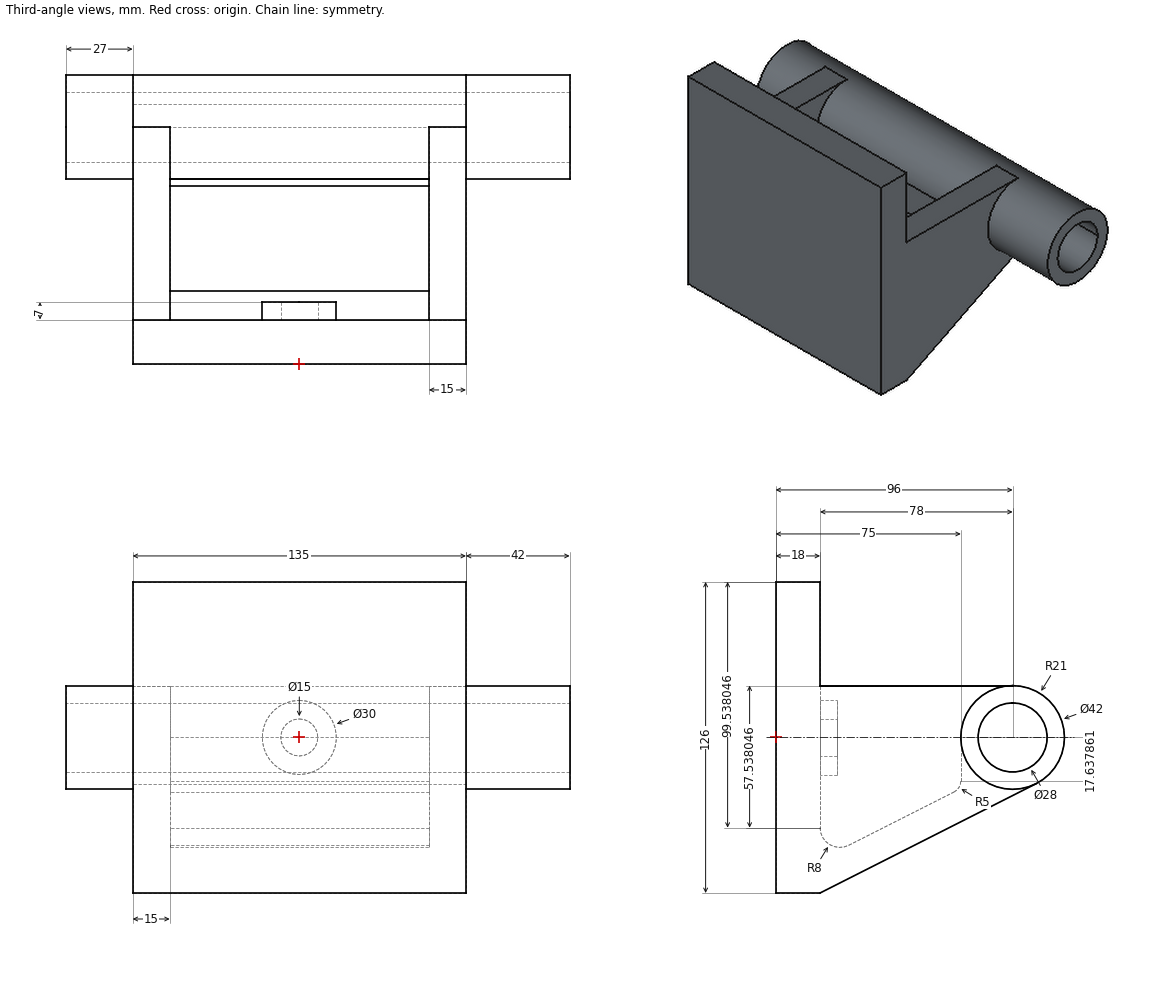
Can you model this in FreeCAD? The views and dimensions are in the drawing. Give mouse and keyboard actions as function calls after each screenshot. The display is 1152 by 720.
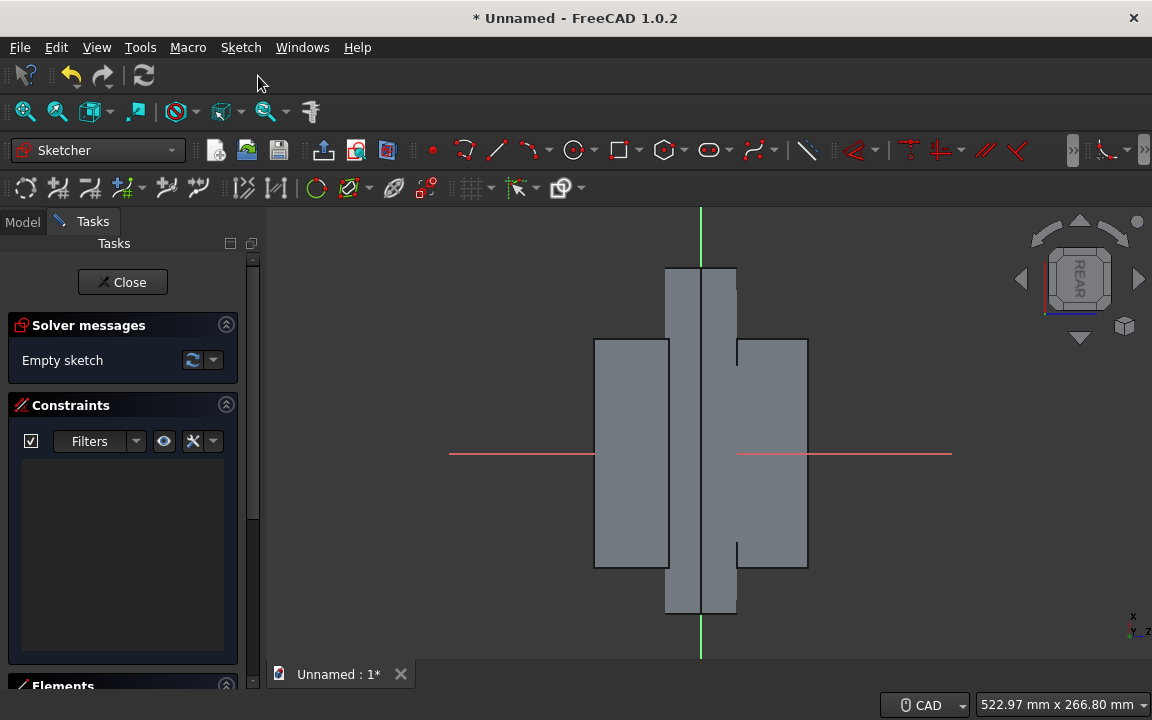
scroll(713, 458, up, 9)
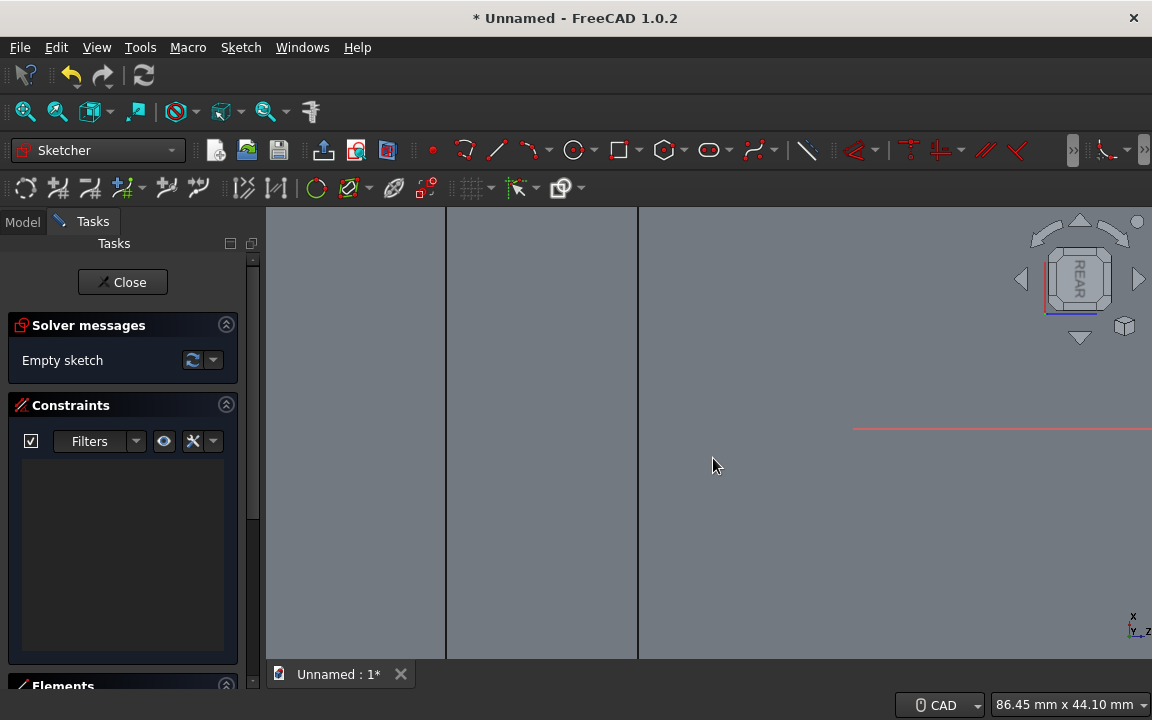
click(574, 150)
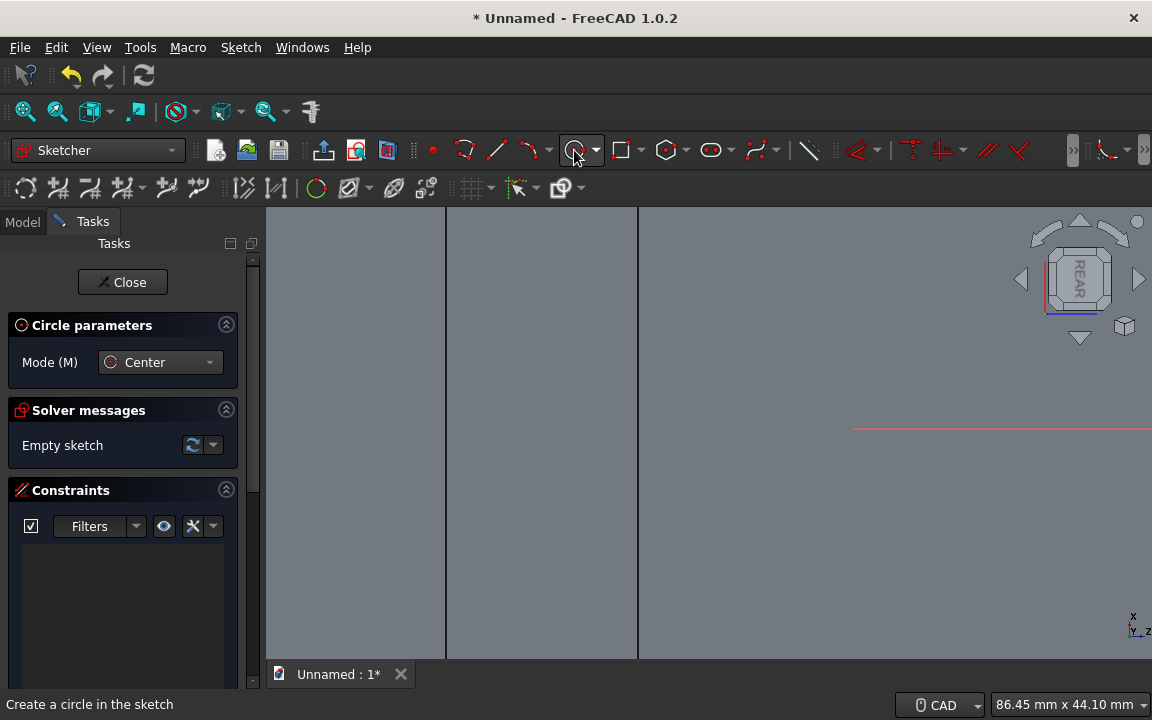
click(638, 429)
click(746, 321)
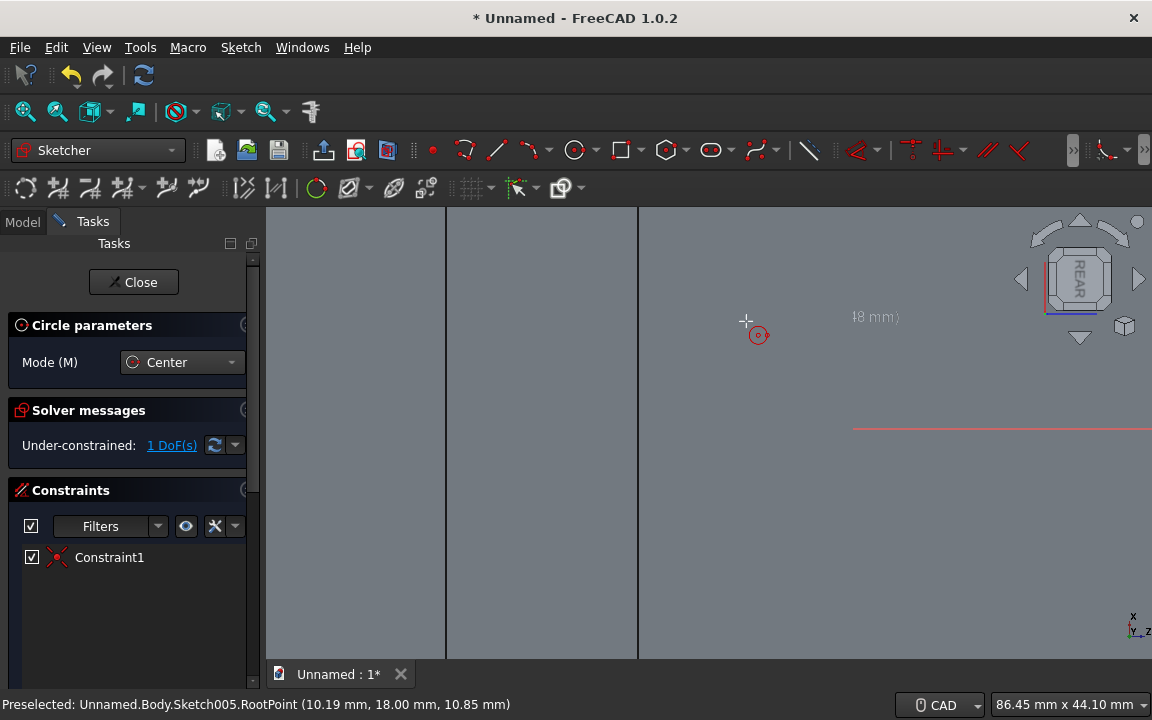
click(638, 429)
click(692, 375)
key(Escape)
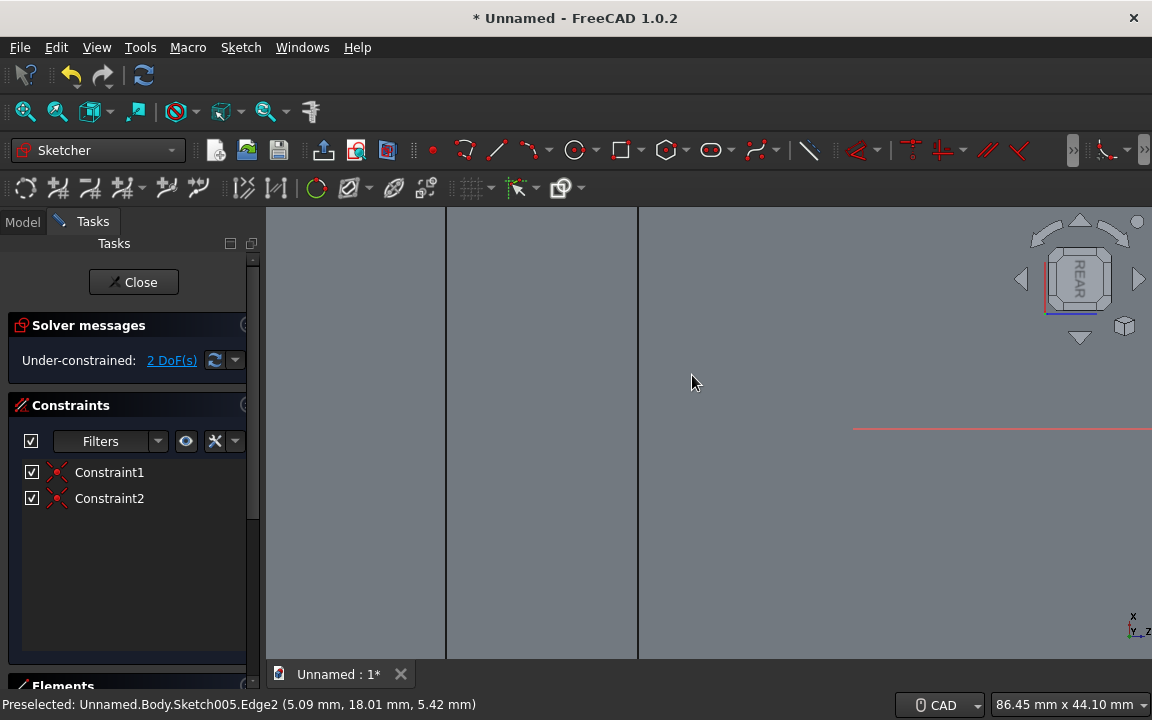
click(856, 150)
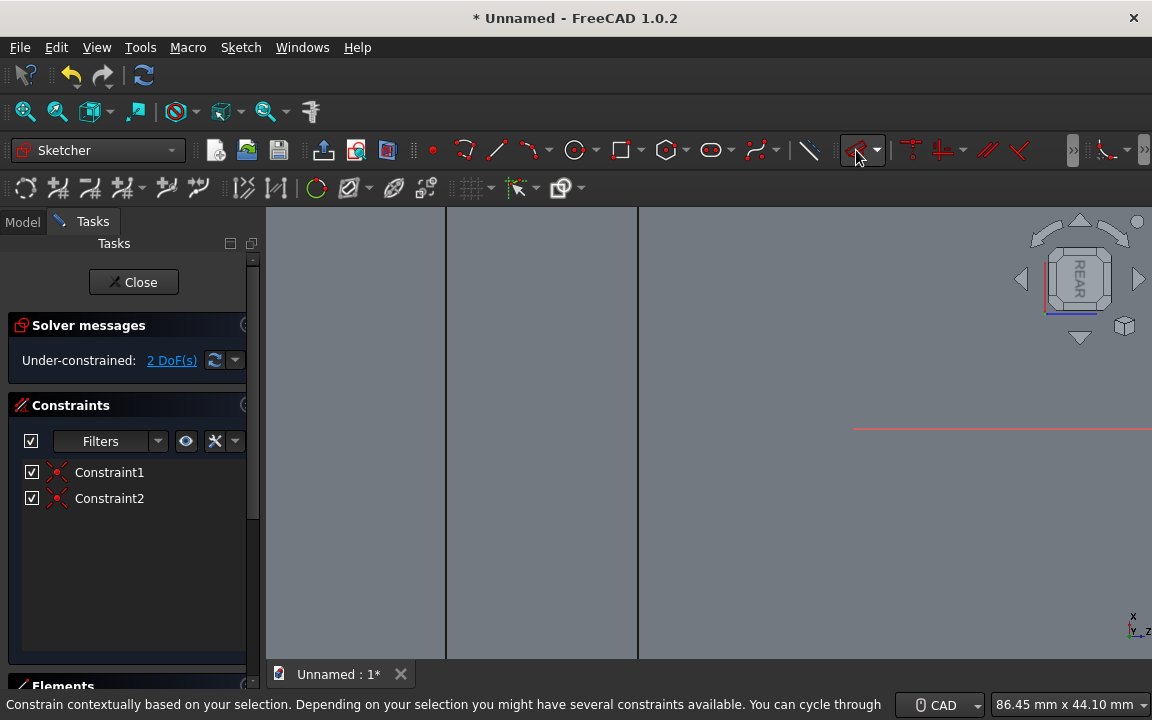
click(745, 321)
click(768, 298)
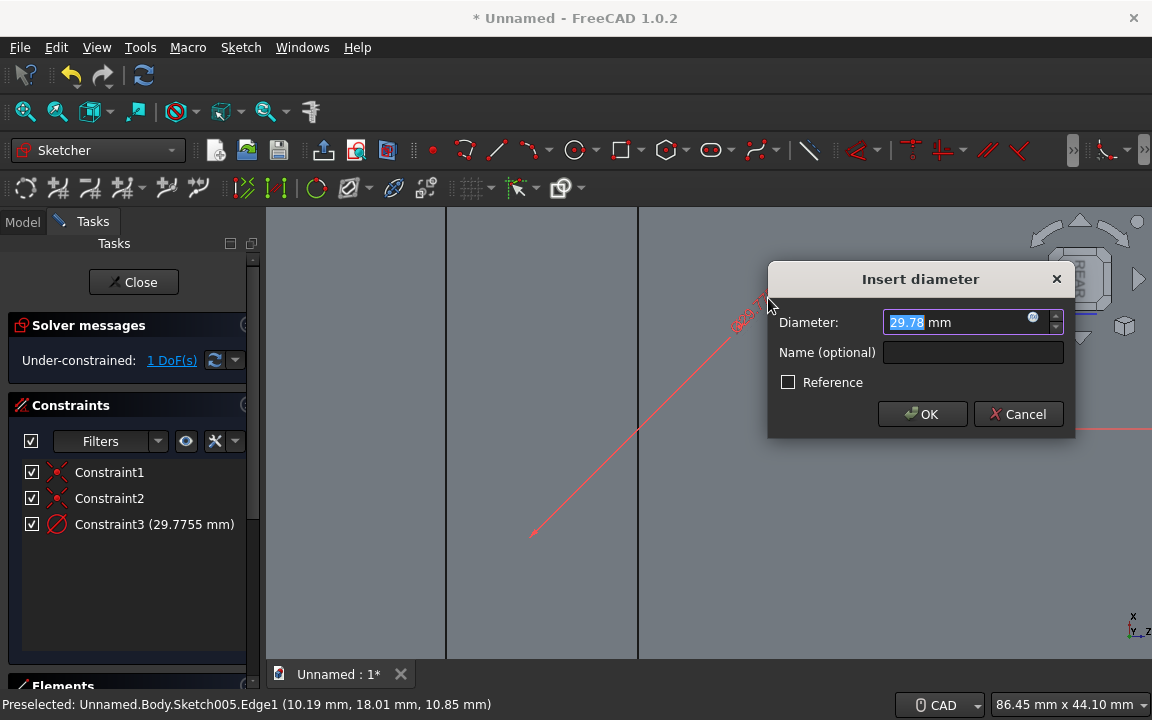
text(30)
key(Return)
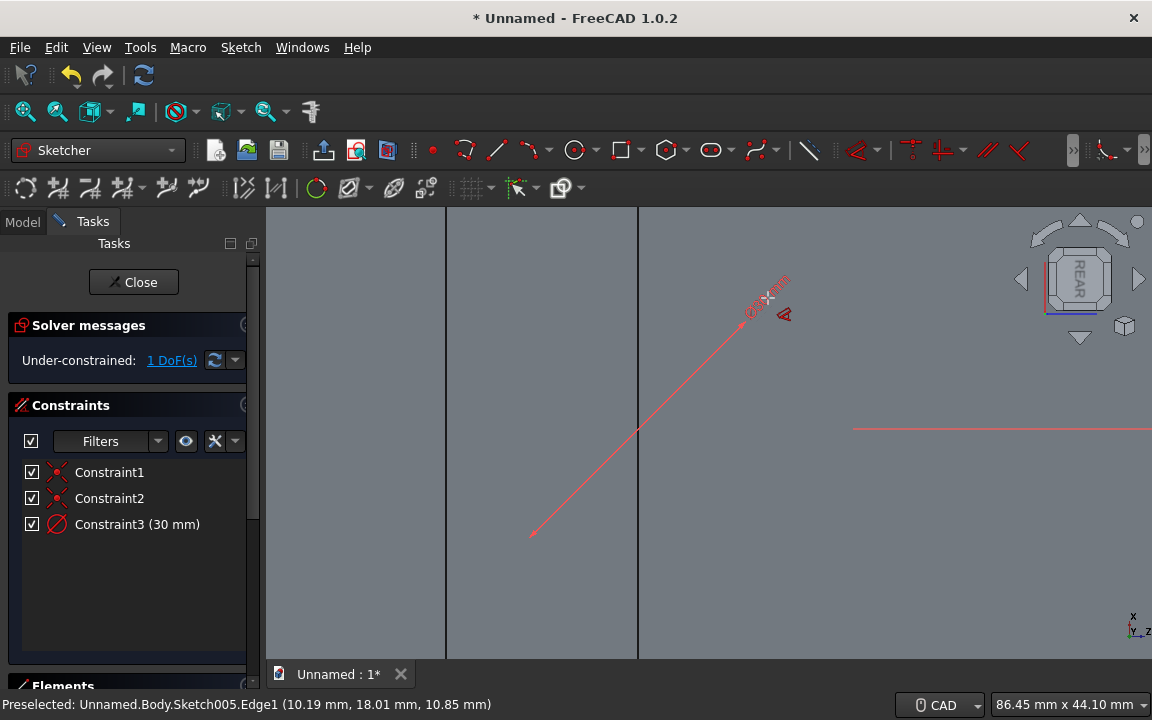
click(691, 375)
click(713, 352)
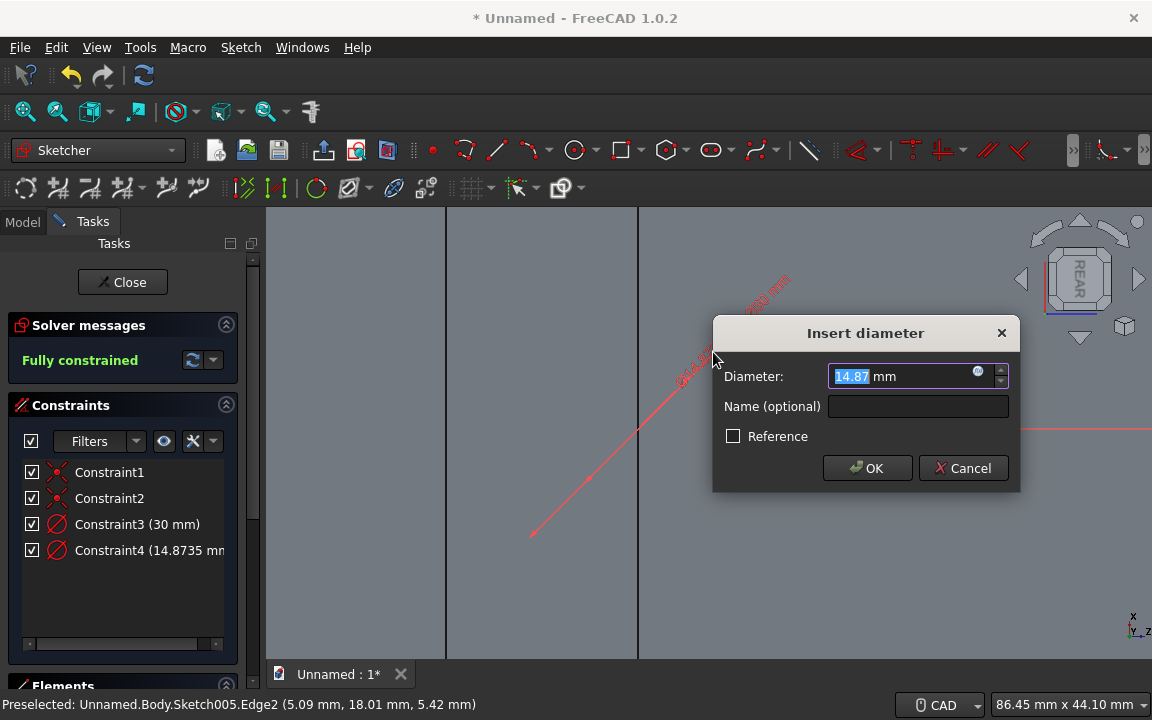
text(15)
key(Return)
key(Escape)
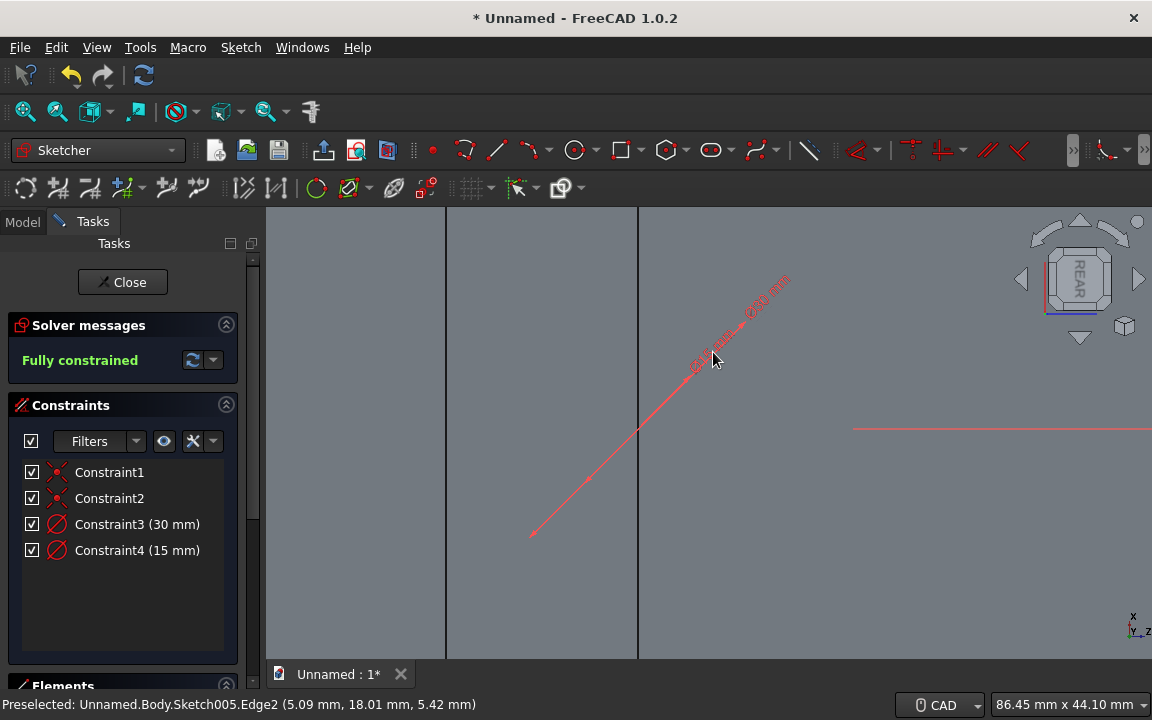
click(123, 282)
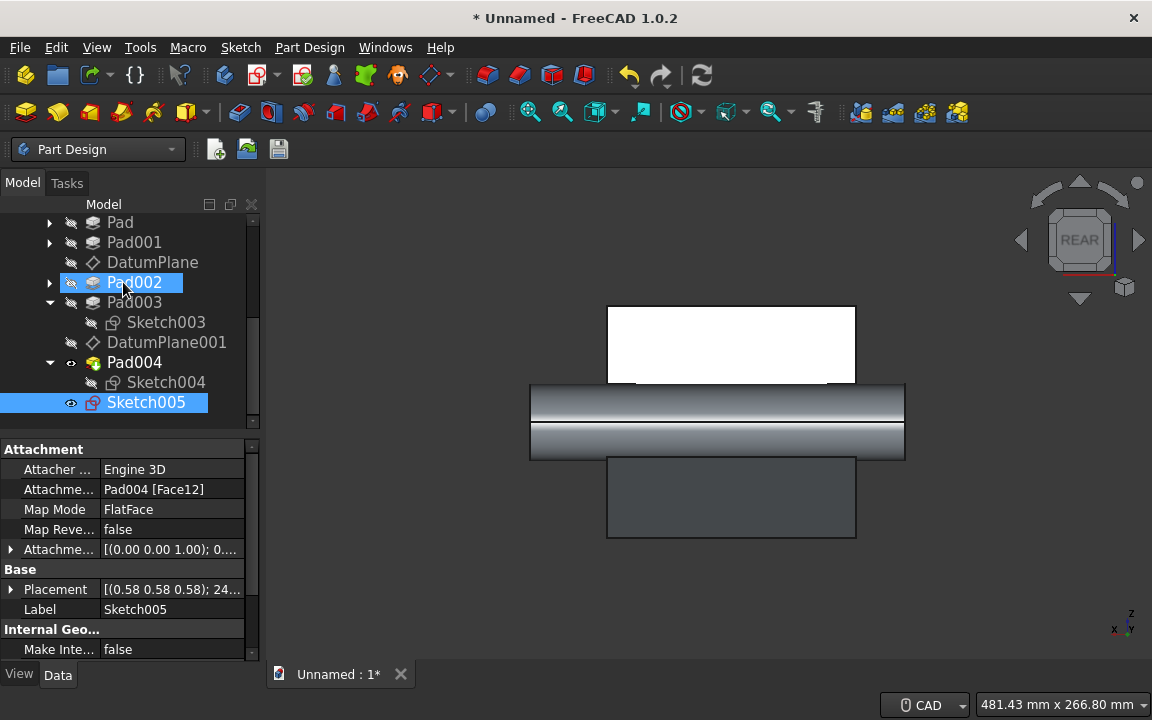
click(26, 112)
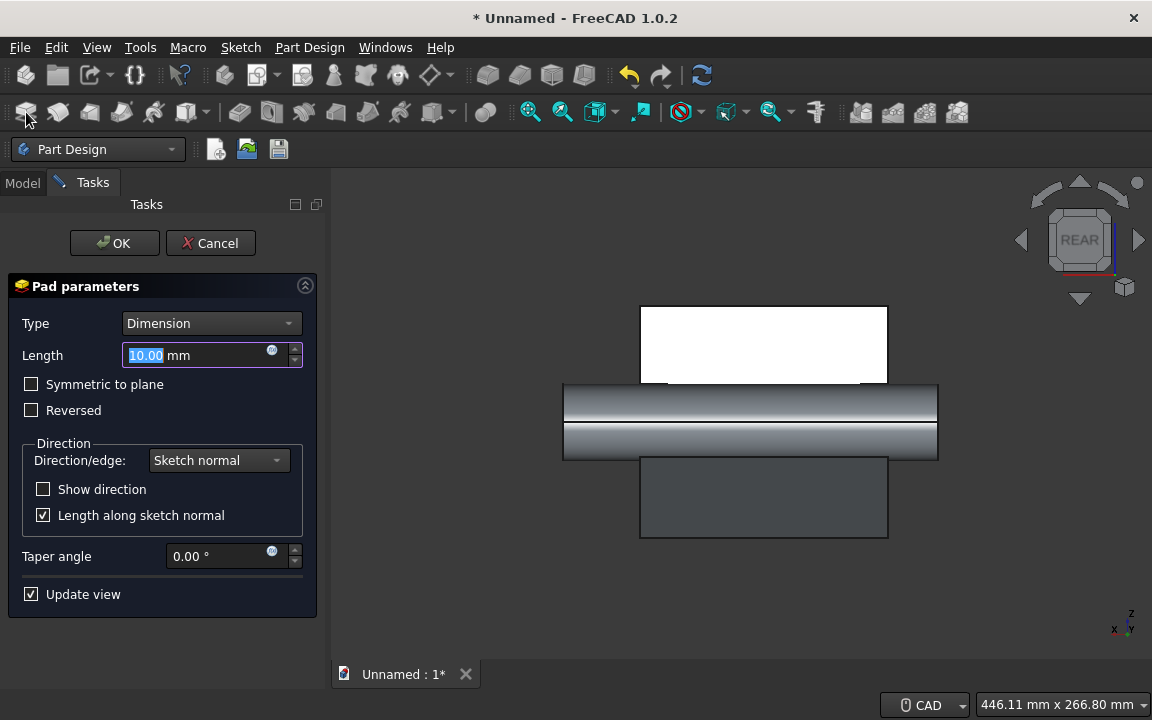
text(7)
key(Tab)